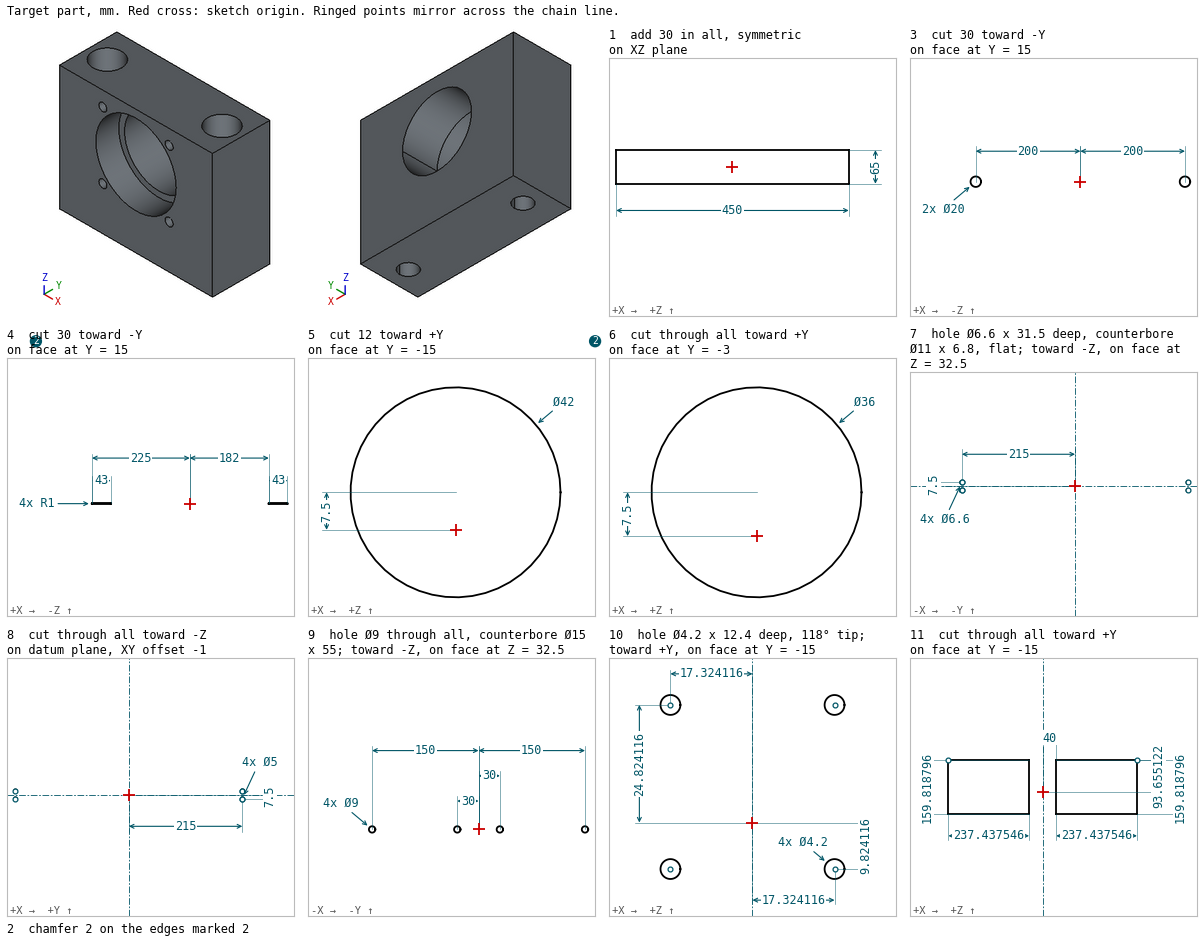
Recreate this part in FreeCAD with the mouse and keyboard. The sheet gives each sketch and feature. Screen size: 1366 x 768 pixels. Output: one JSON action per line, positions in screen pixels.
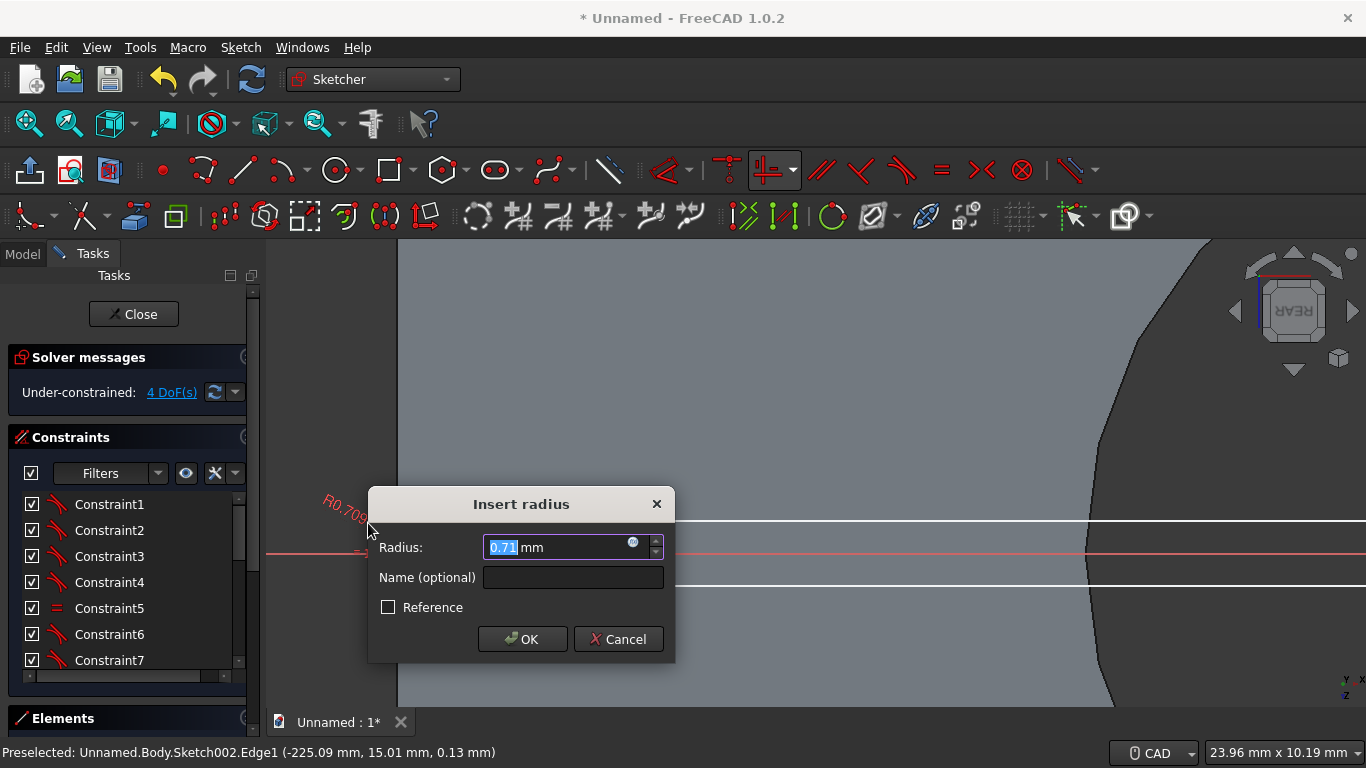
{"action": "type", "text": "1"}
{"action": "key", "text": "Return"}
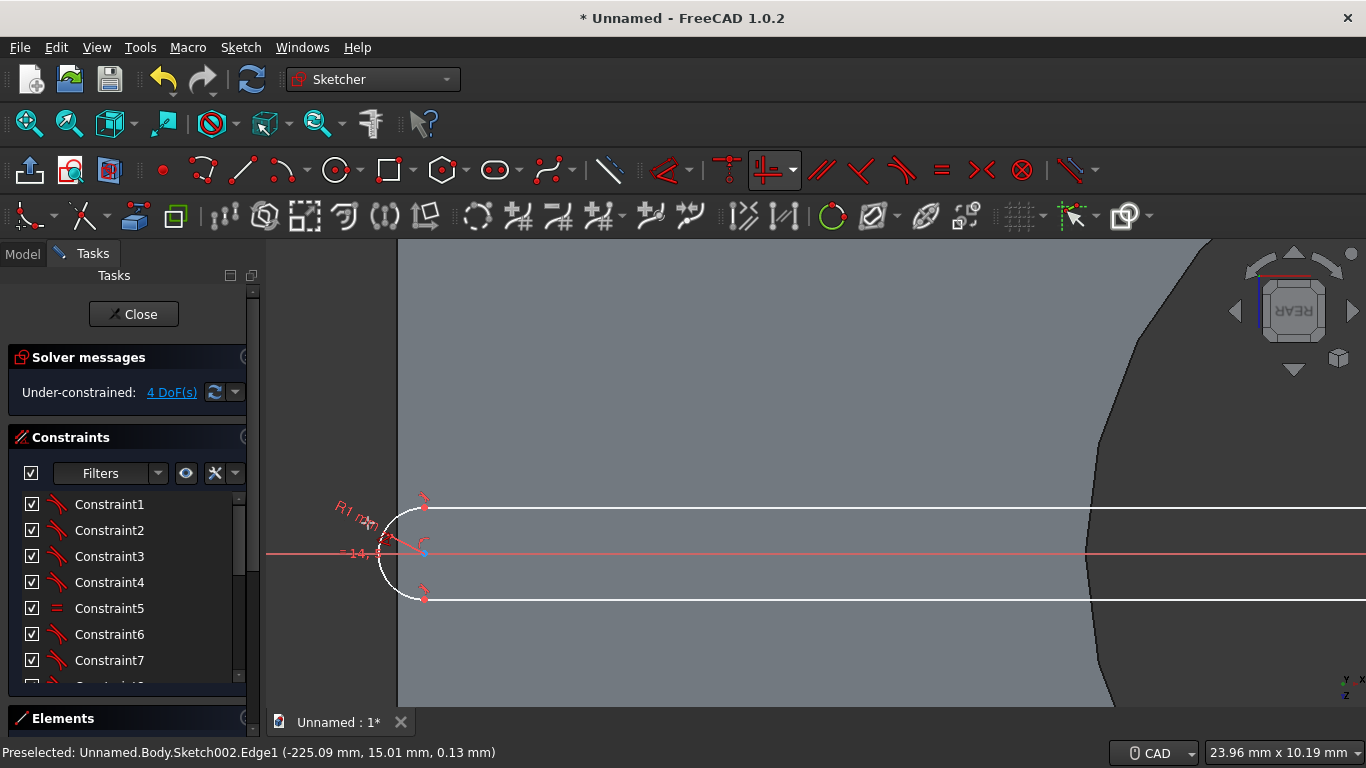
{"action": "scroll", "coordinate": [323, 470], "scroll_direction": "down", "scroll_amount": 16}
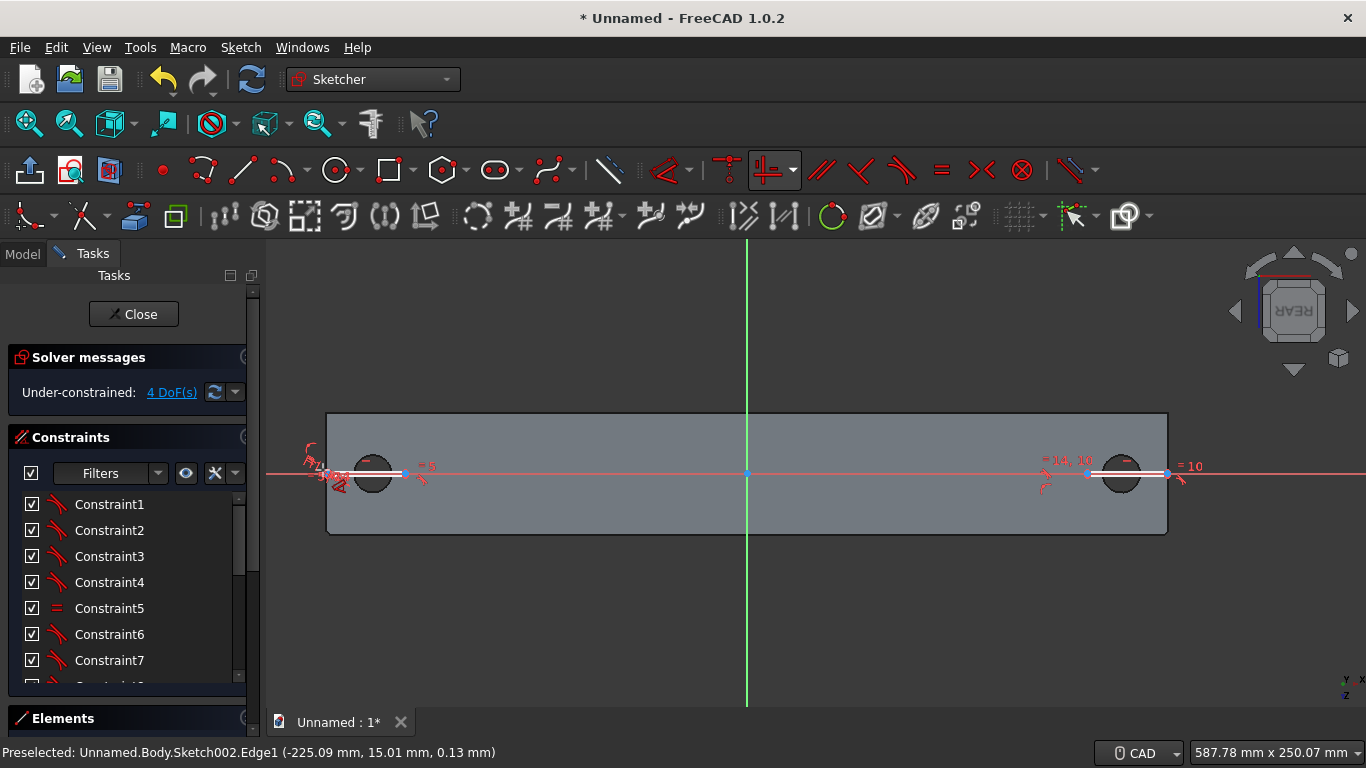
{"action": "scroll", "coordinate": [351, 472], "scroll_direction": "up", "scroll_amount": 10}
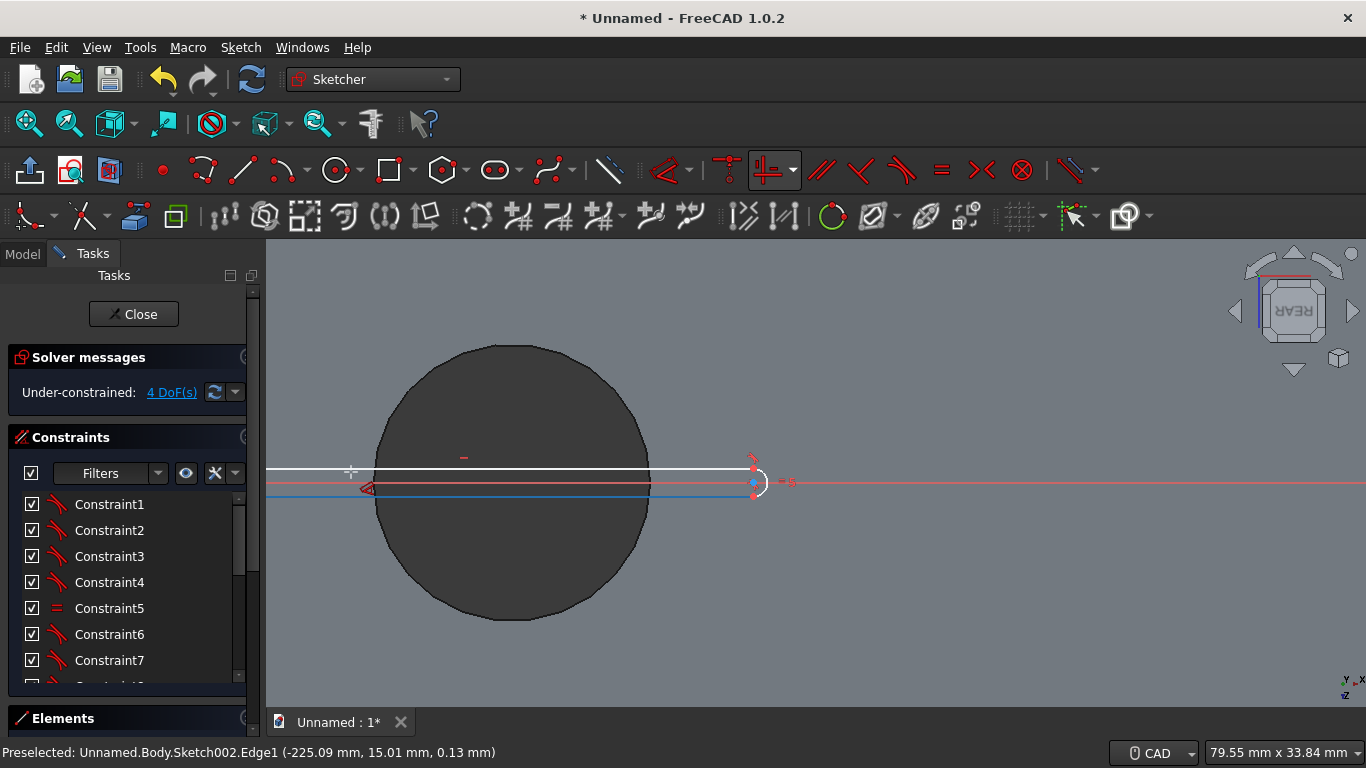
{"action": "left_click", "coordinate": [348, 469]}
{"action": "left_click", "coordinate": [524, 435]}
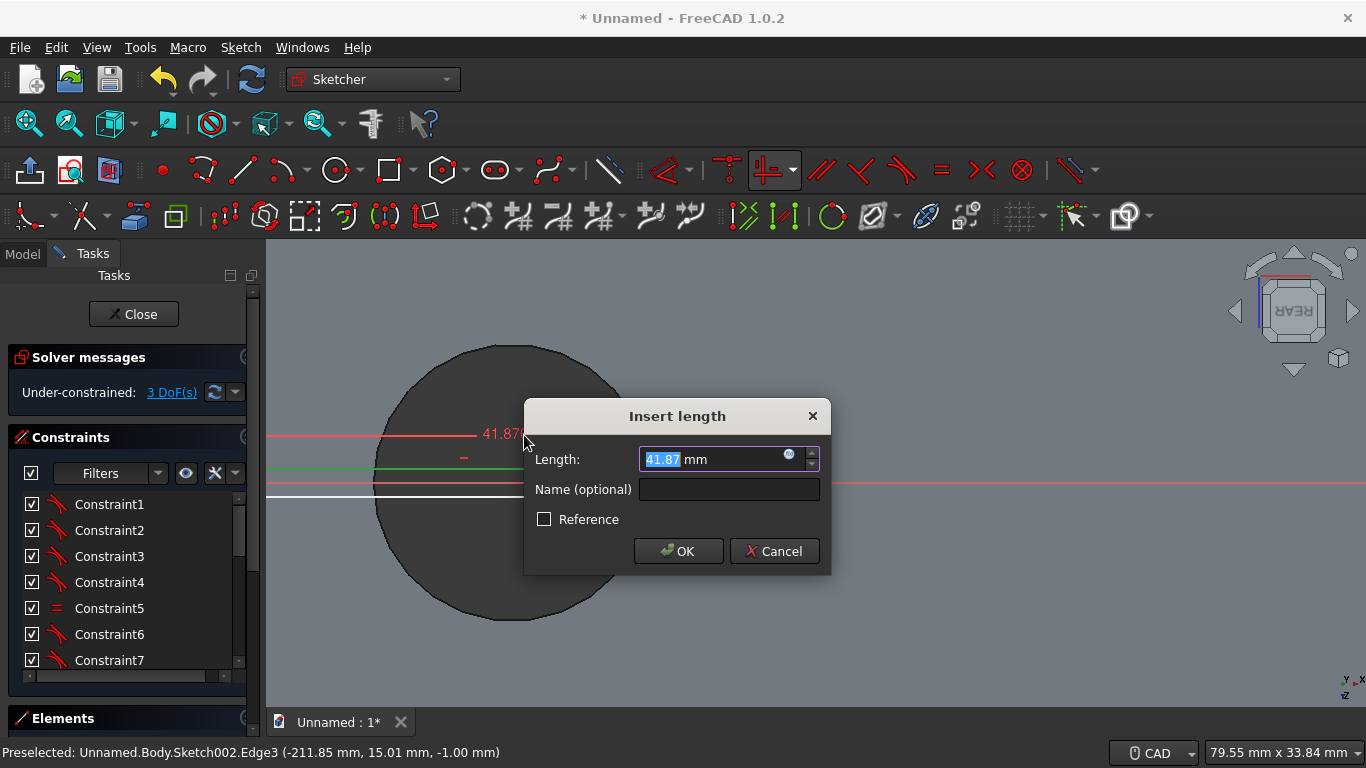
{"action": "type", "text": "43"}
{"action": "key", "text": "Return"}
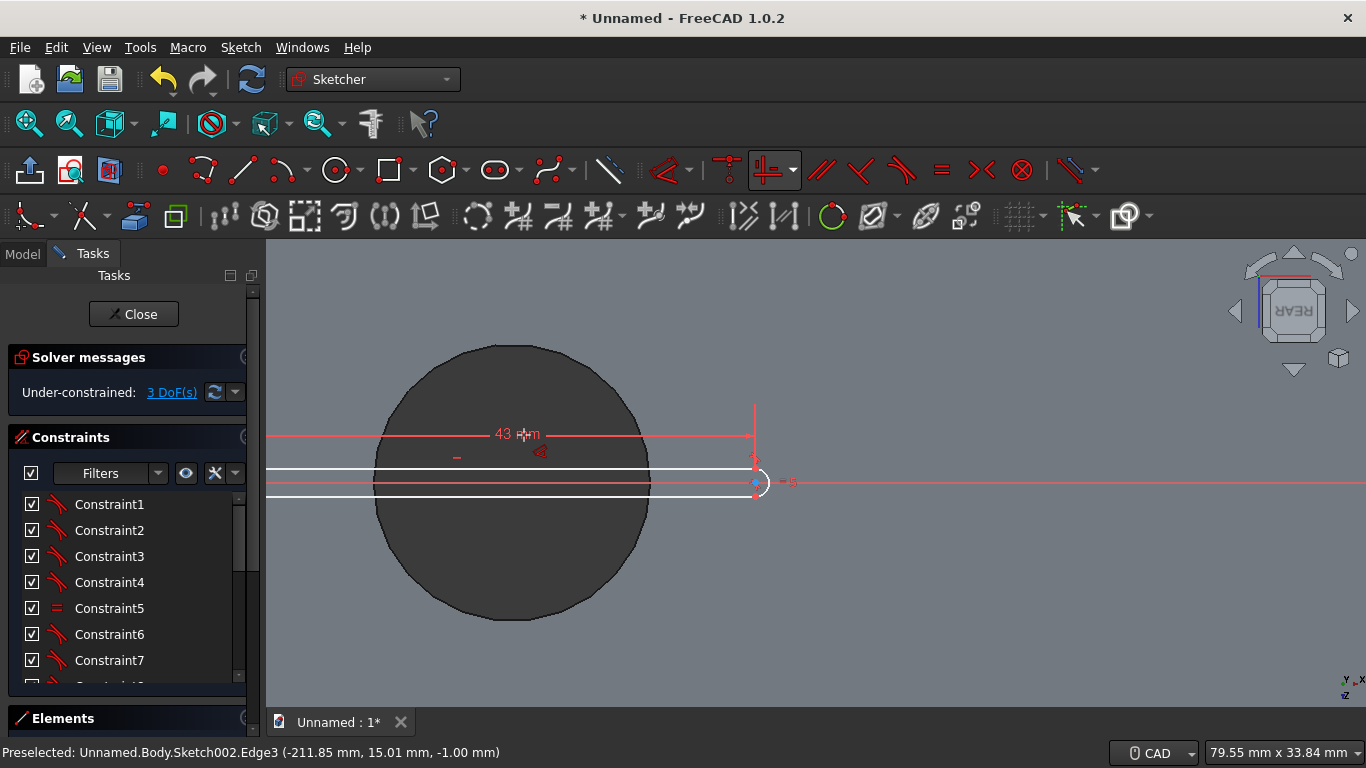
{"action": "scroll", "coordinate": [432, 472], "scroll_direction": "down", "scroll_amount": 11}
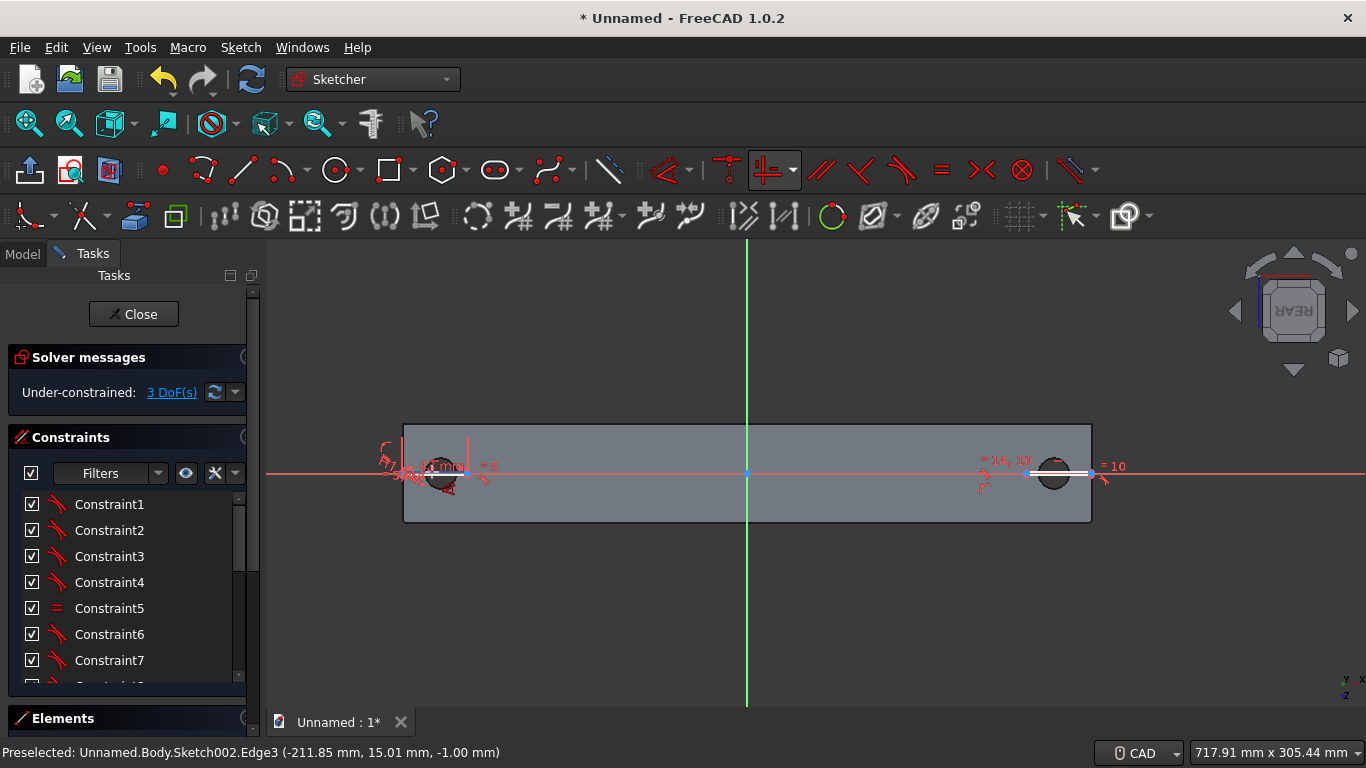
{"action": "scroll", "coordinate": [1046, 472], "scroll_direction": "up", "scroll_amount": 11}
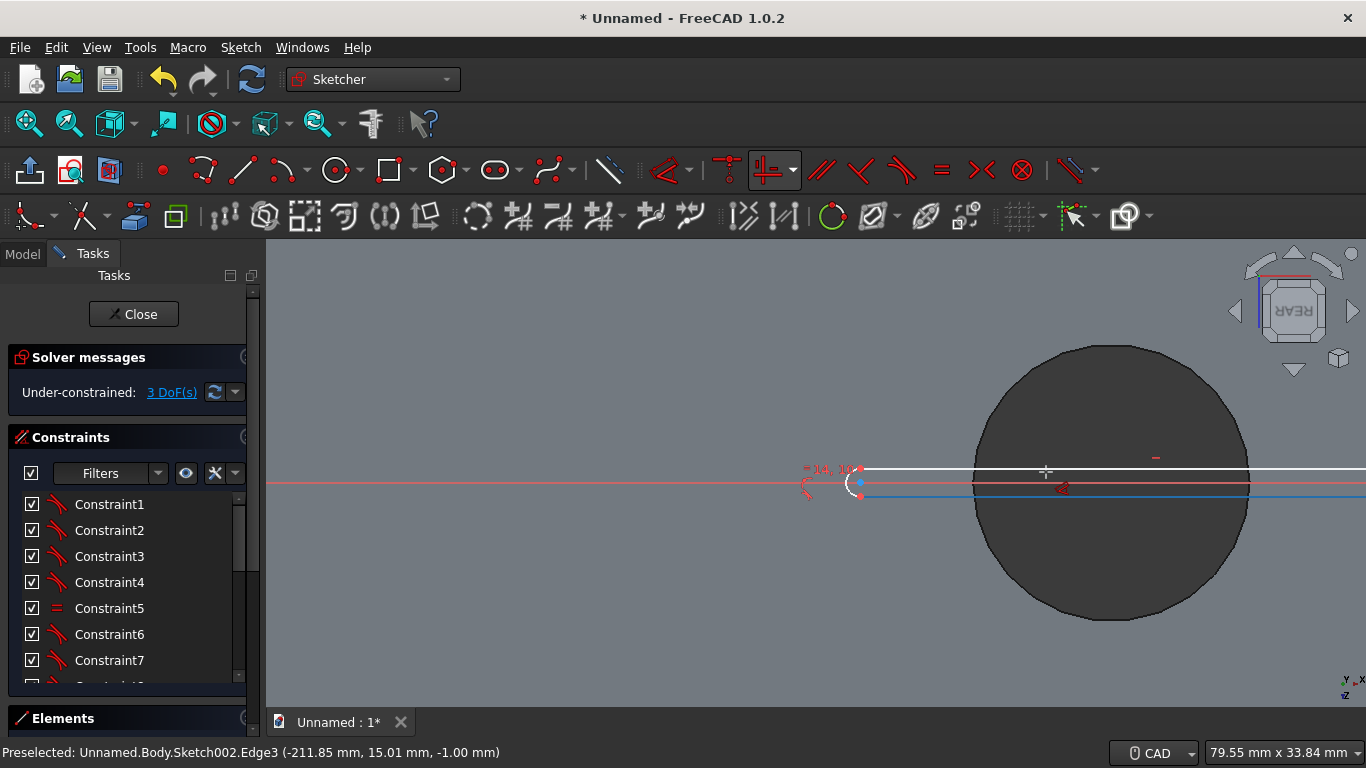
{"action": "left_click", "coordinate": [1038, 469]}
{"action": "left_click", "coordinate": [1031, 435]}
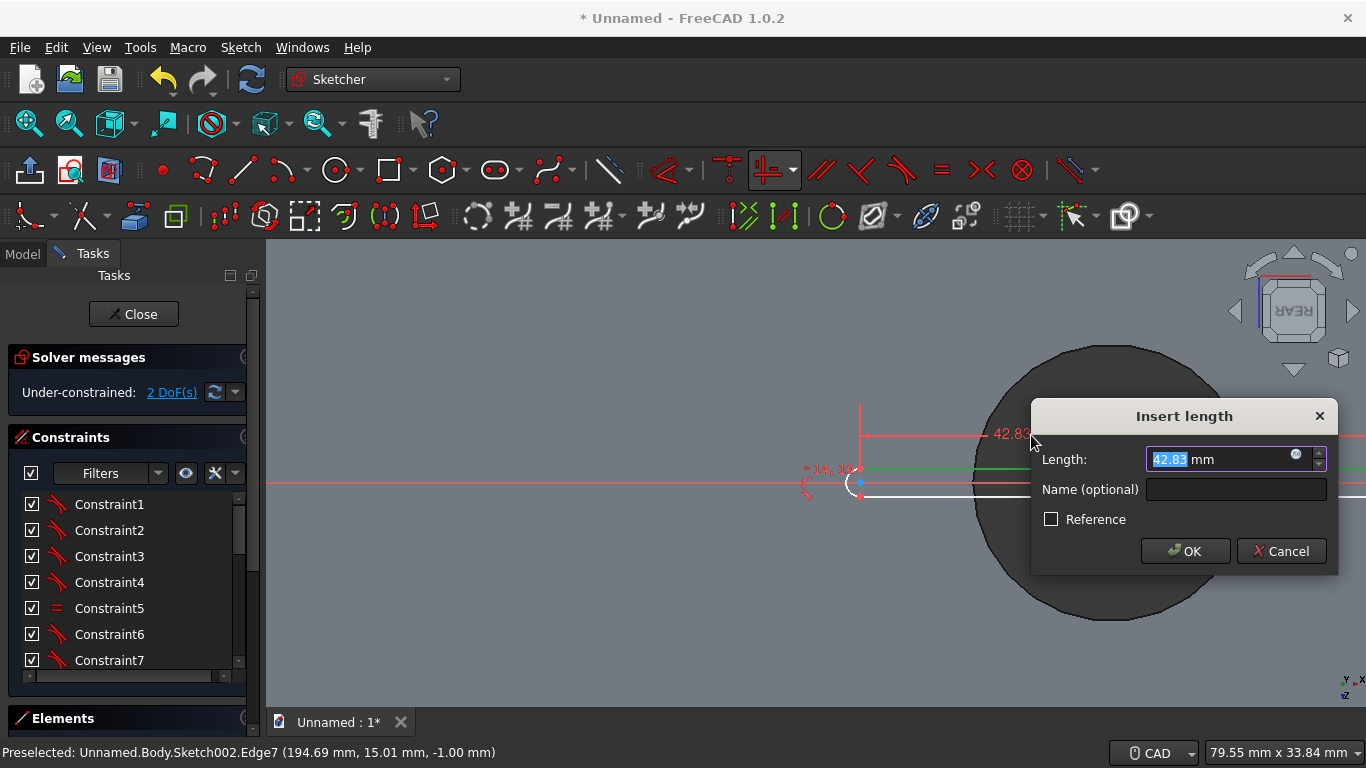
{"action": "type", "text": "43"}
{"action": "key", "text": "Return"}